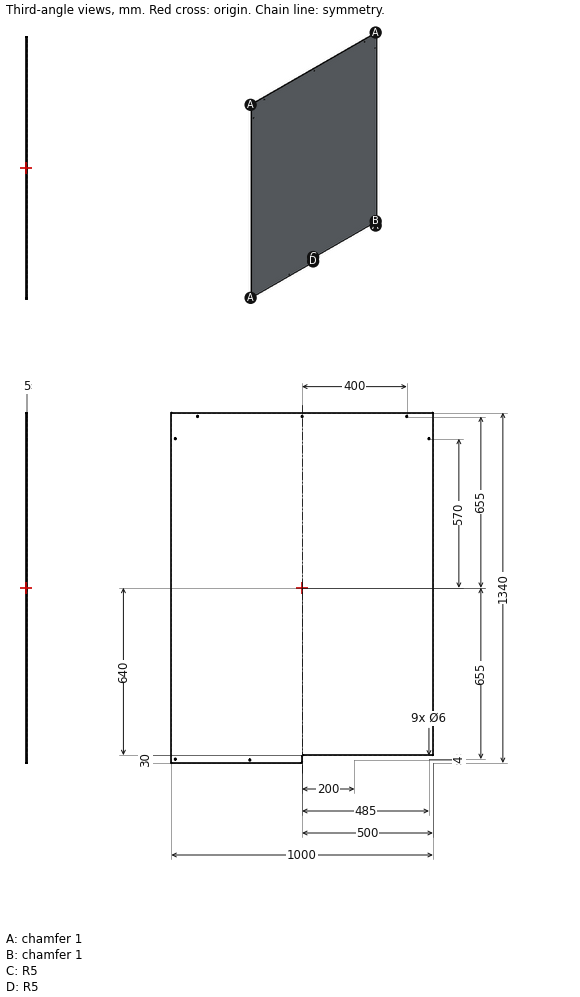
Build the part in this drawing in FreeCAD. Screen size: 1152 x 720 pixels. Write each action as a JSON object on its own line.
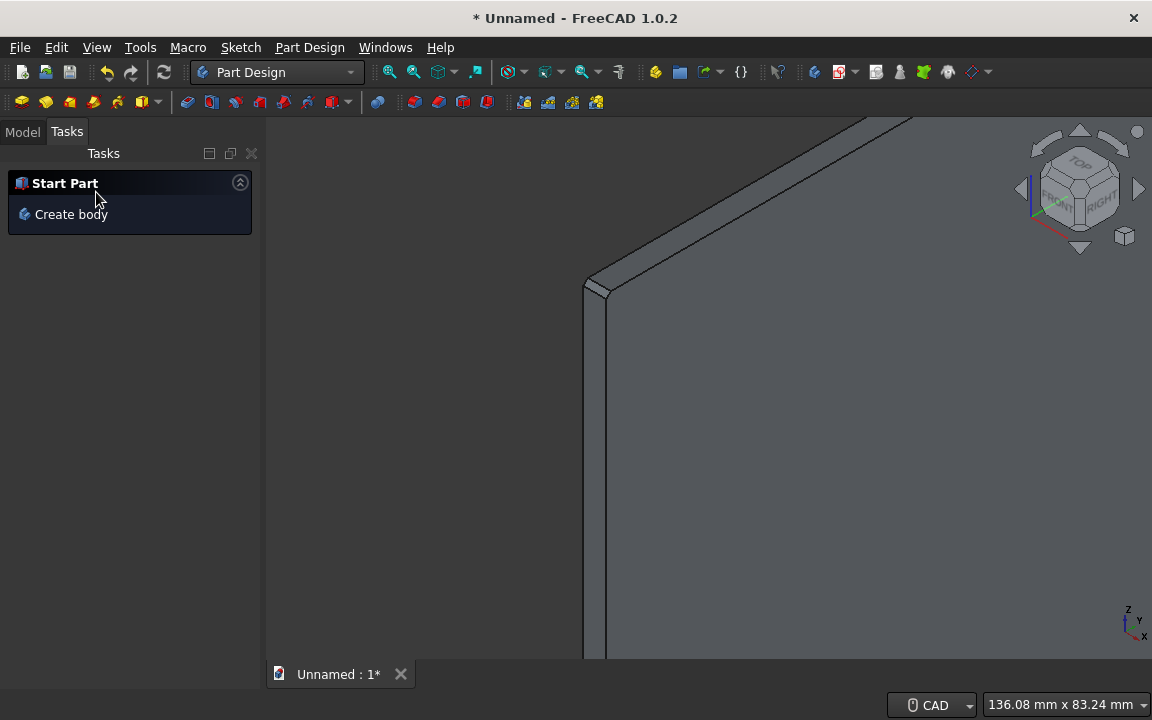
{"action": "left_click", "coordinate": [390, 72]}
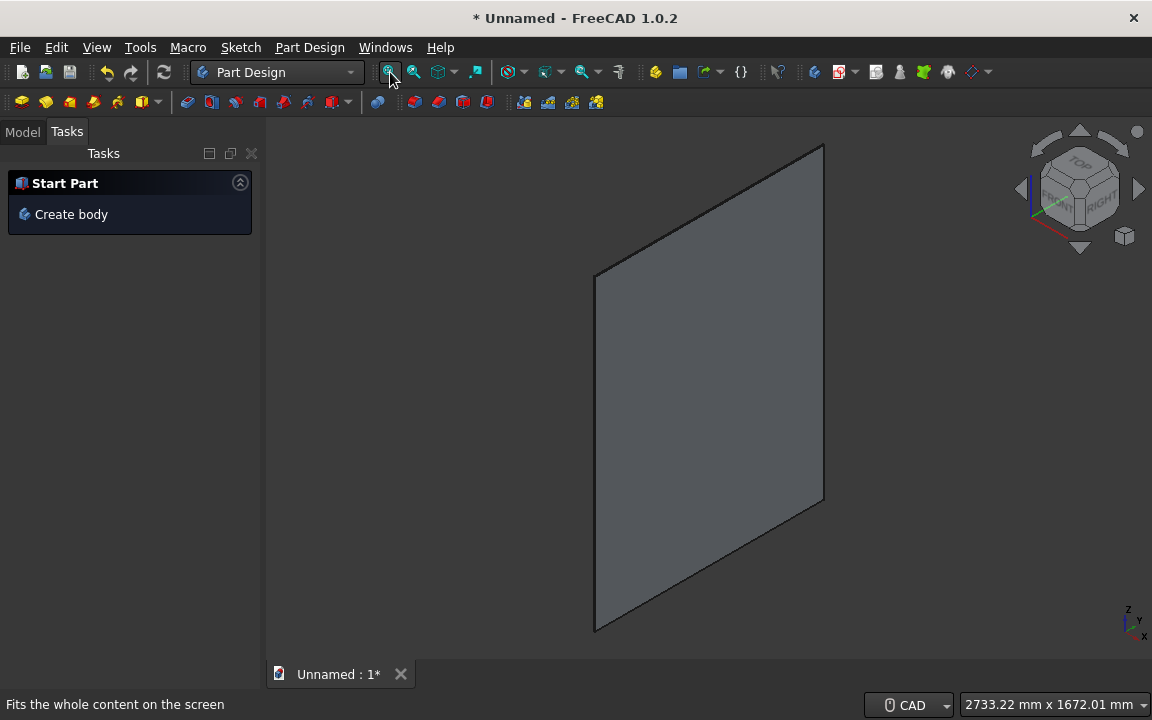
{"action": "left_click", "coordinate": [840, 72]}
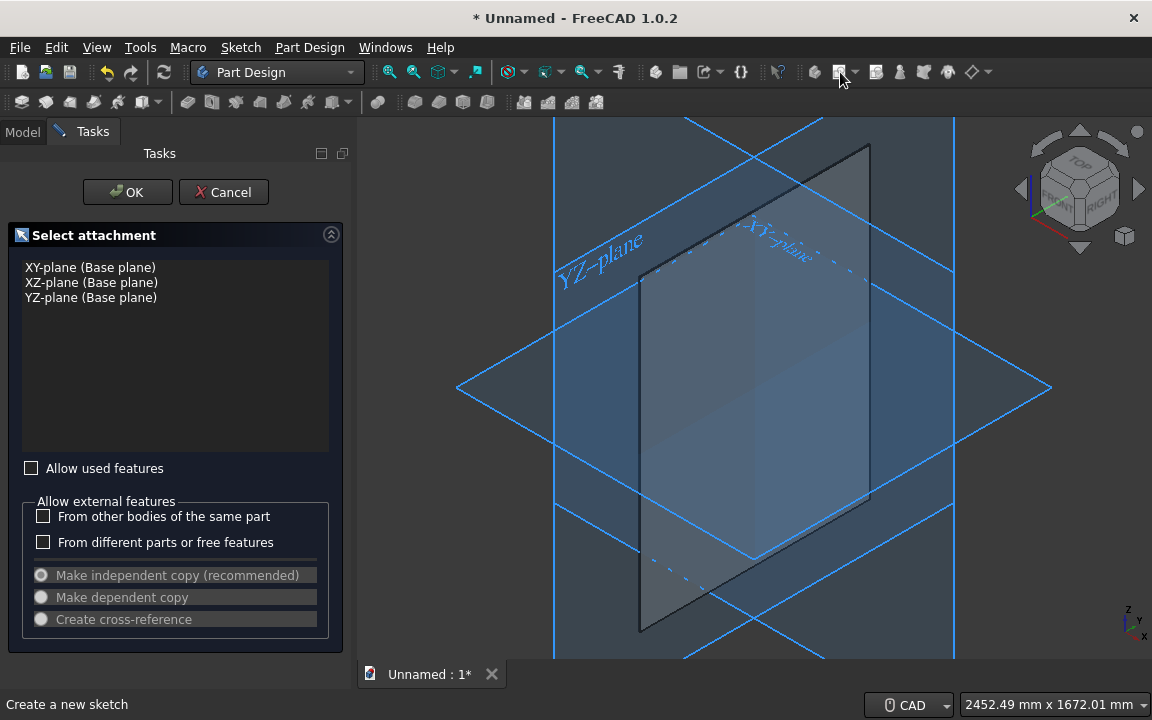
{"action": "left_click", "coordinate": [82, 298]}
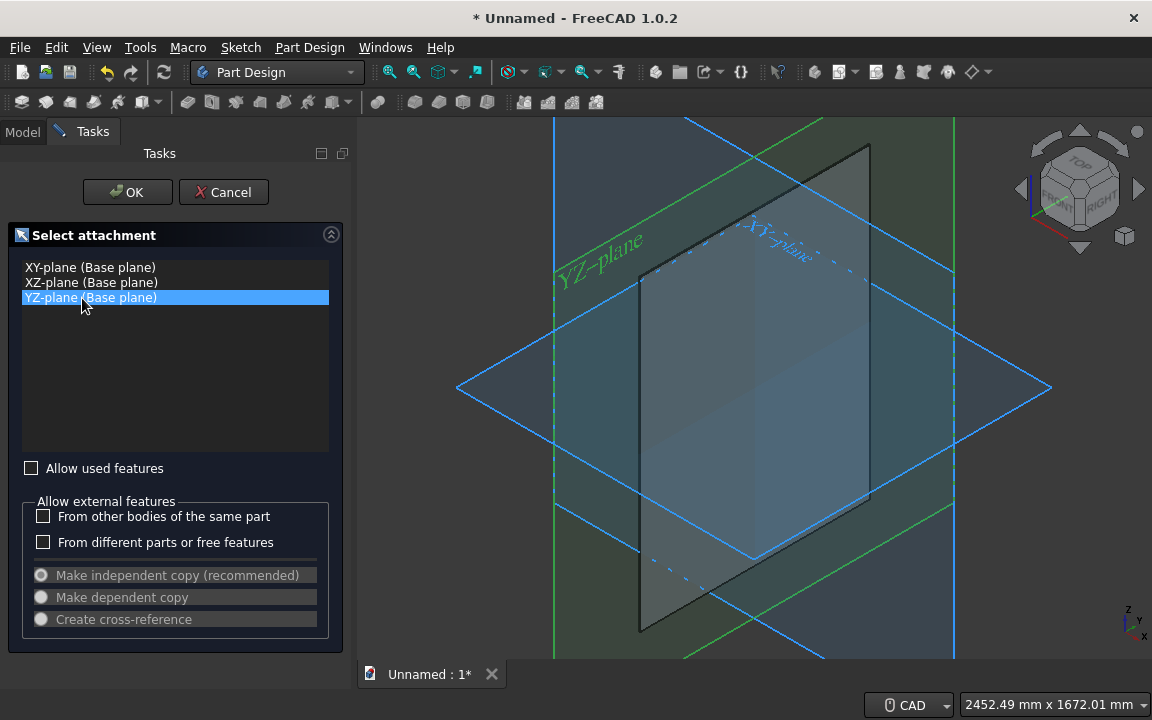
{"action": "left_click", "coordinate": [128, 192]}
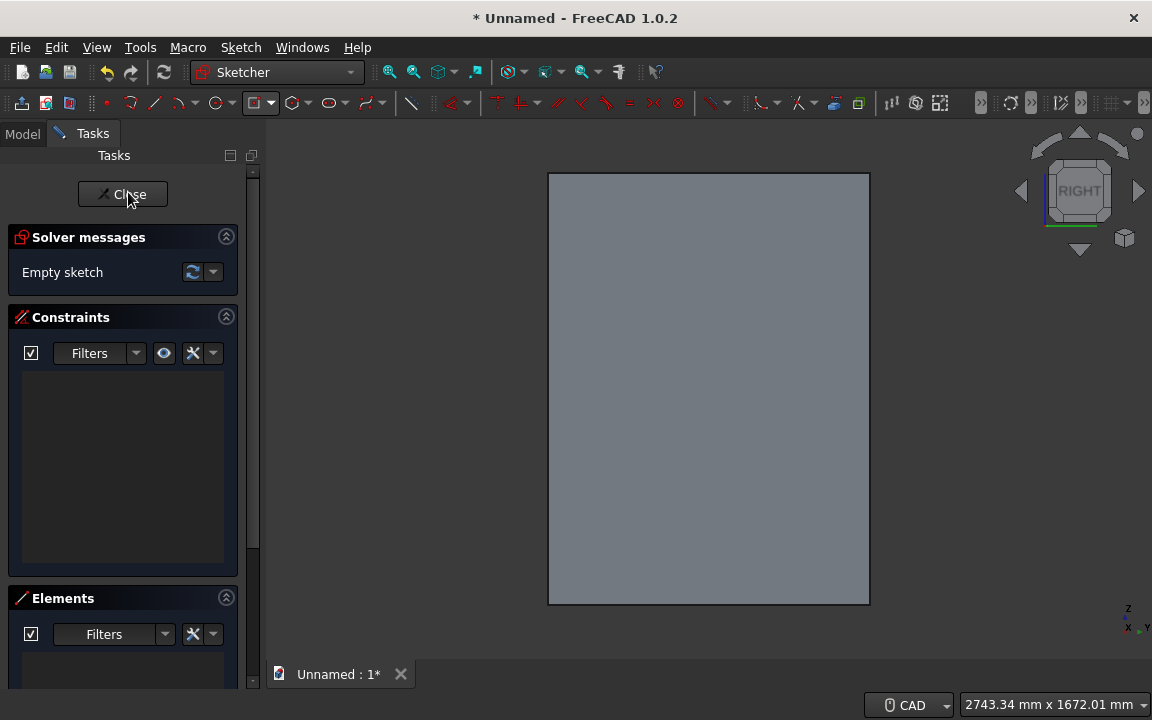
{"action": "left_click", "coordinate": [70, 104]}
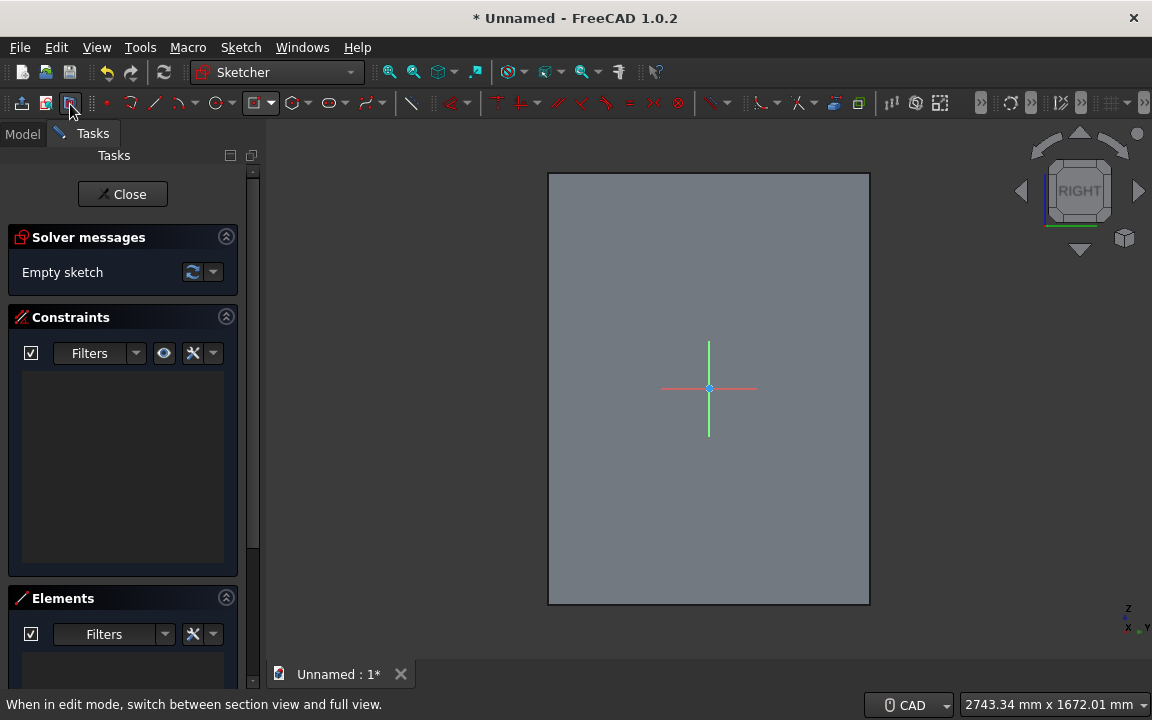
{"action": "left_click", "coordinate": [216, 104]}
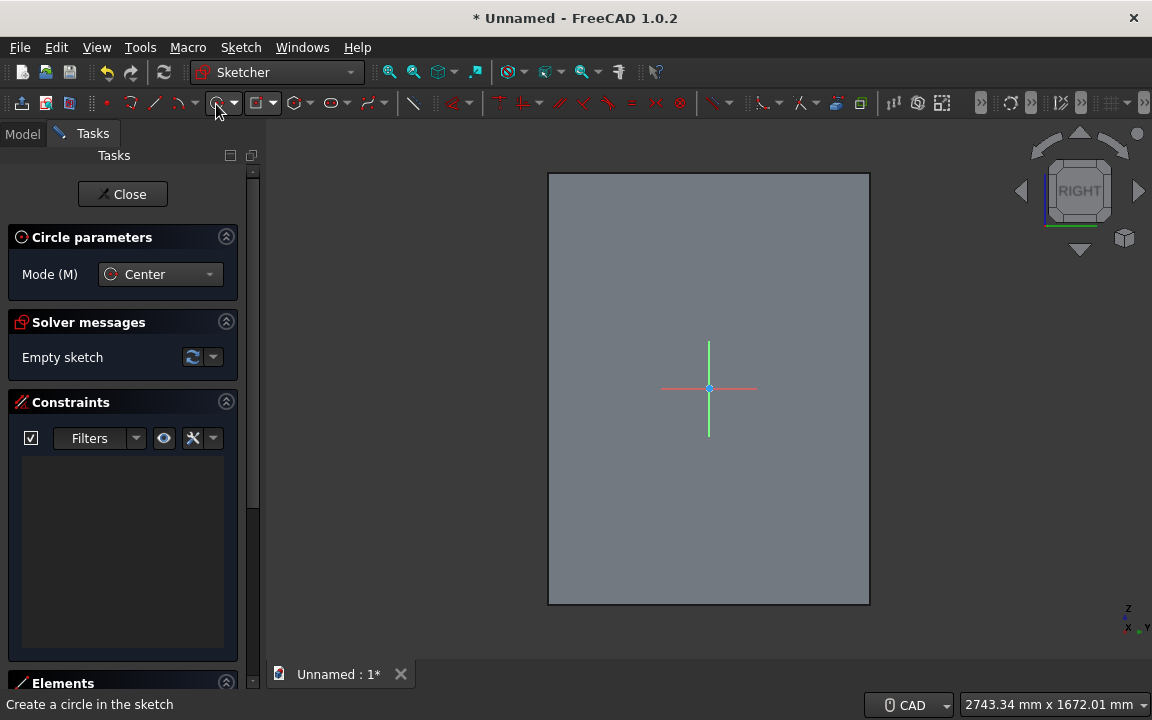
{"action": "scroll", "coordinate": [866, 601], "scroll_direction": "up", "scroll_amount": 16}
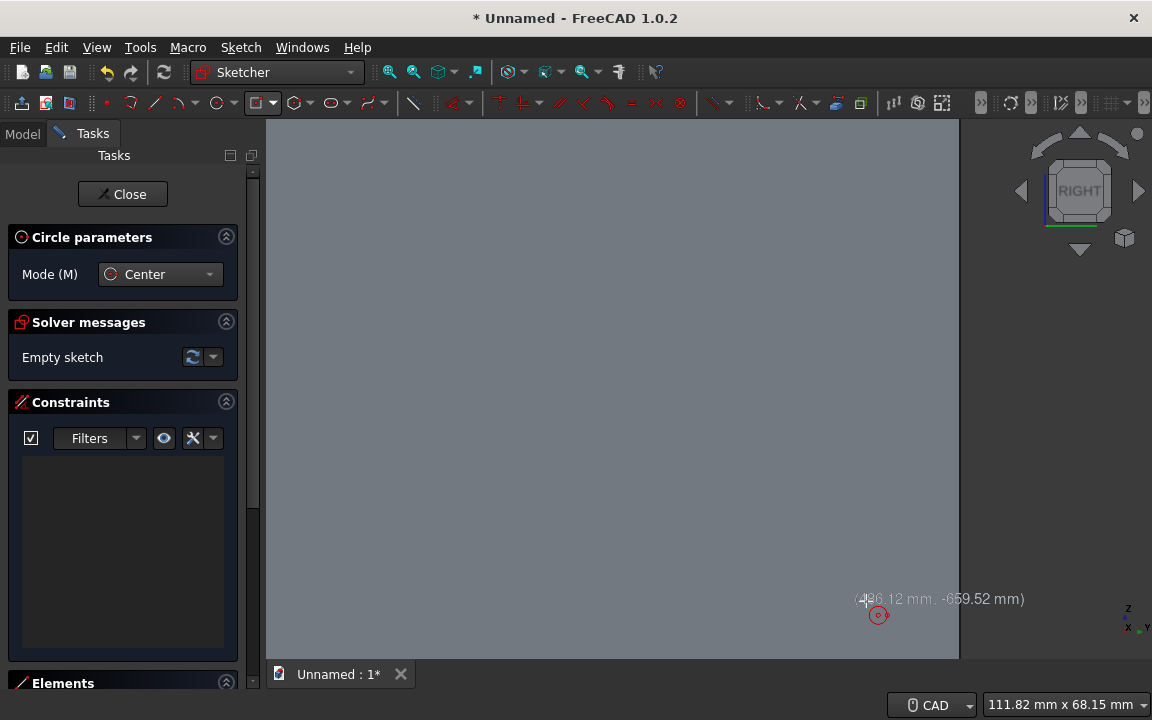
{"action": "scroll", "coordinate": [795, 601], "scroll_direction": "down", "scroll_amount": 16}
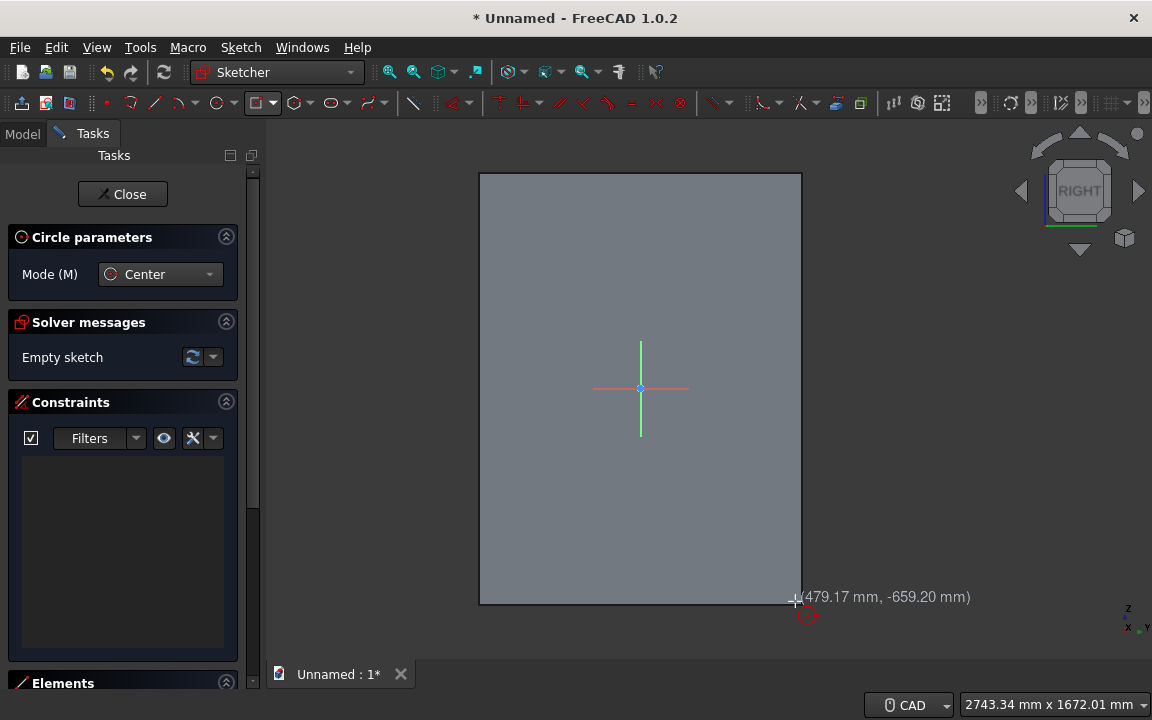
{"action": "left_click", "coordinate": [797, 601]}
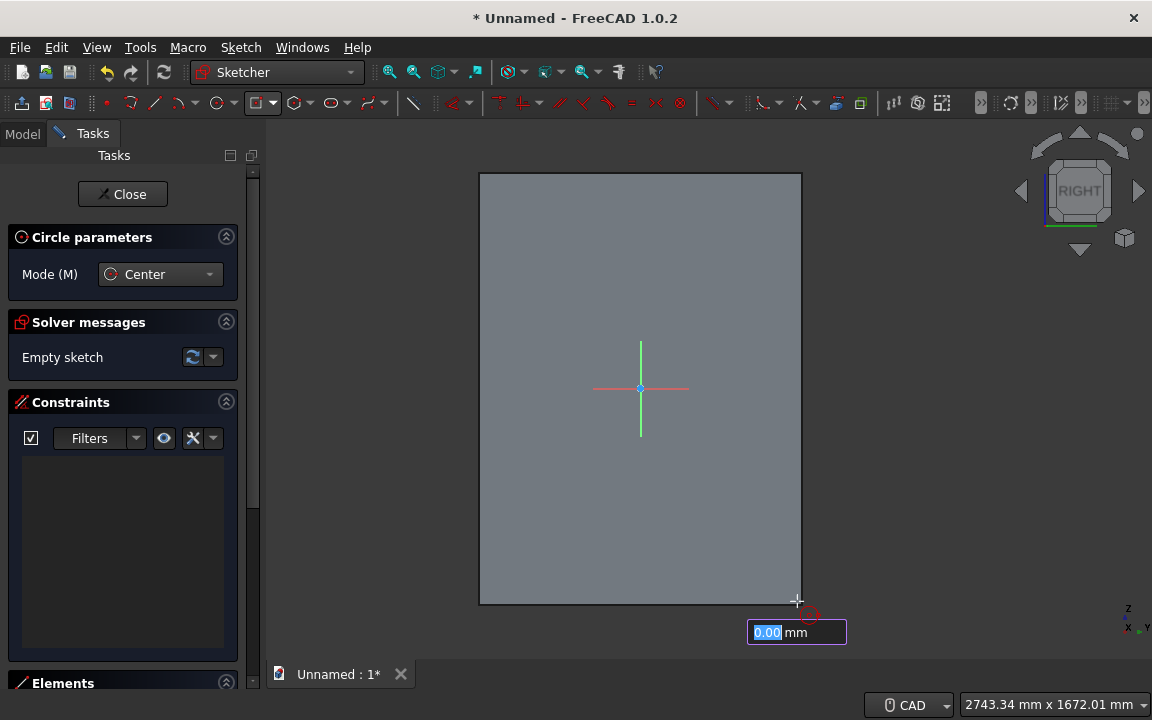
{"action": "scroll", "coordinate": [798, 600], "scroll_direction": "up", "scroll_amount": 14}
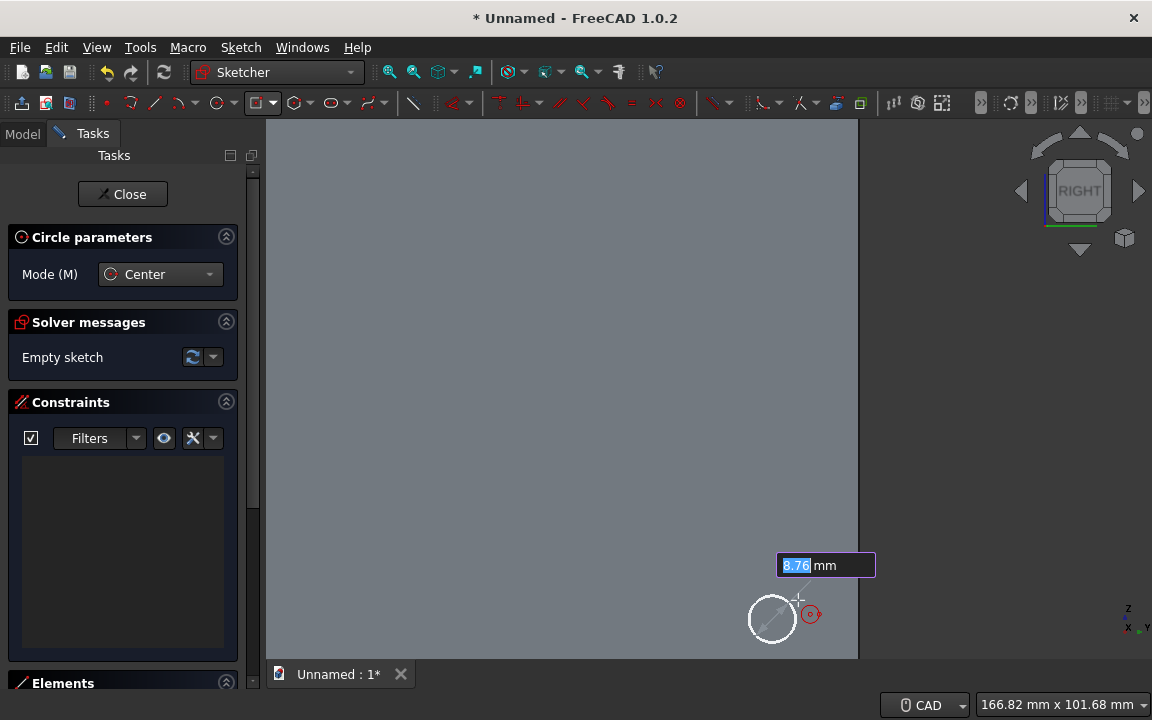
{"action": "left_click", "coordinate": [791, 584]}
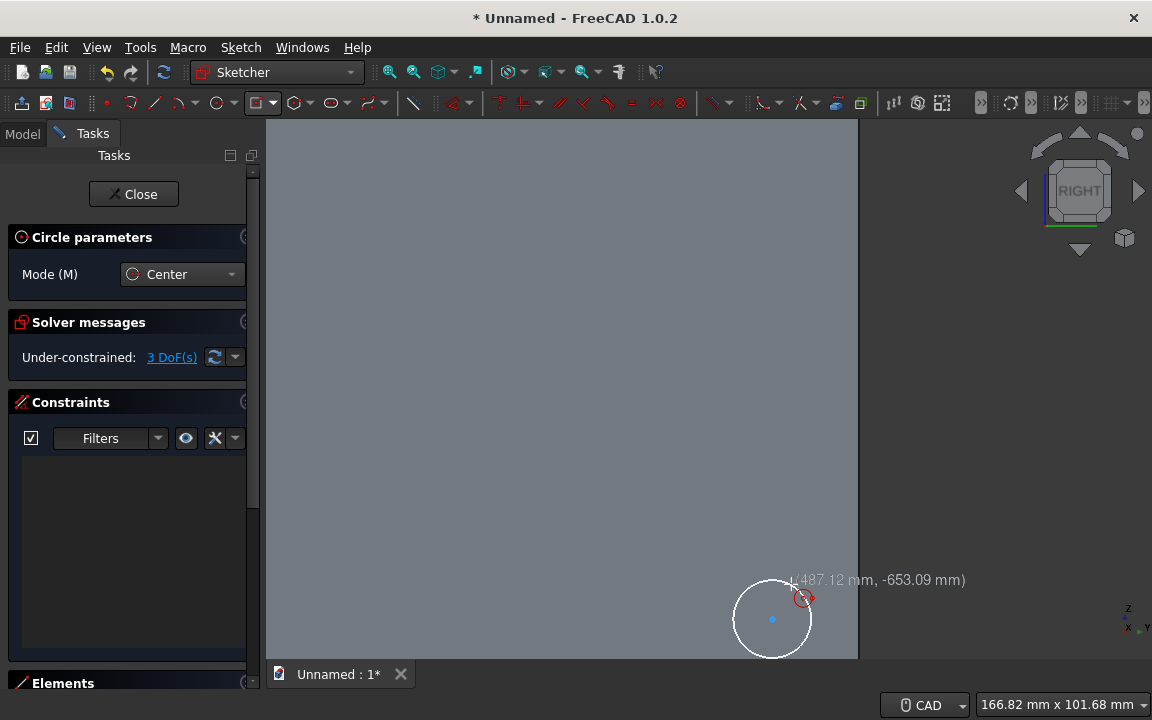
{"action": "scroll", "coordinate": [768, 560], "scroll_direction": "down", "scroll_amount": 15}